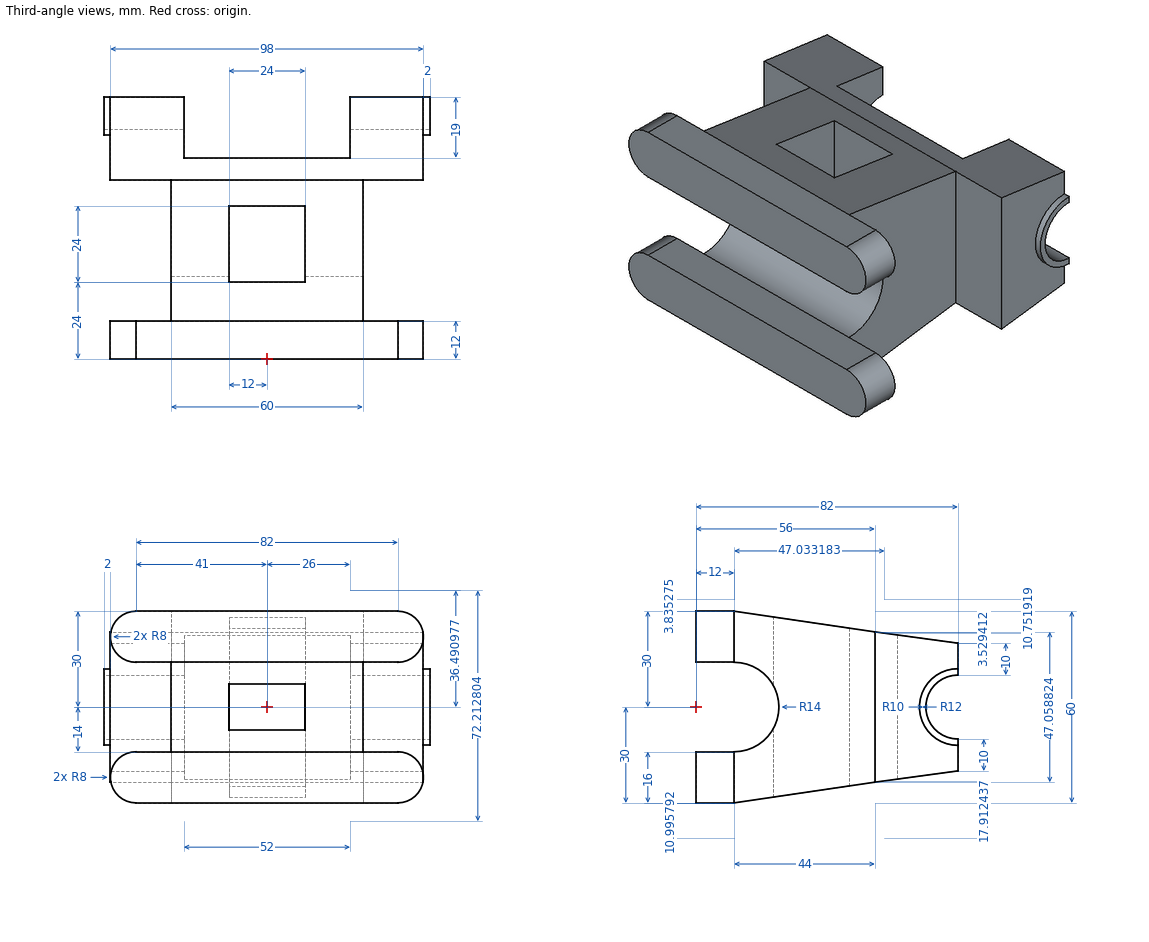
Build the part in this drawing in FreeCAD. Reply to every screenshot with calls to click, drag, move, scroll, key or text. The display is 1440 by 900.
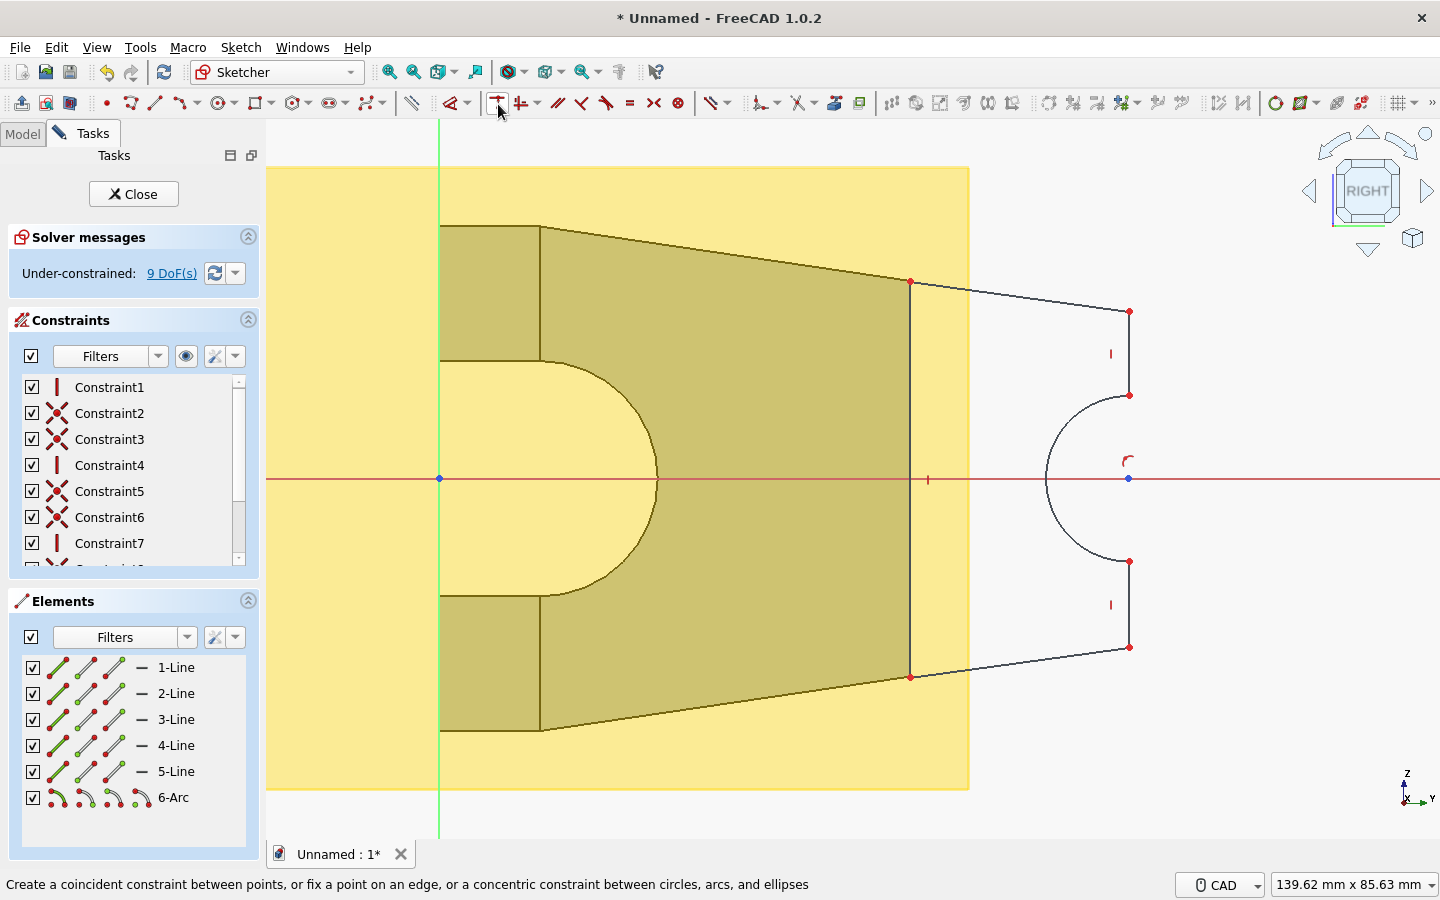
click(450, 104)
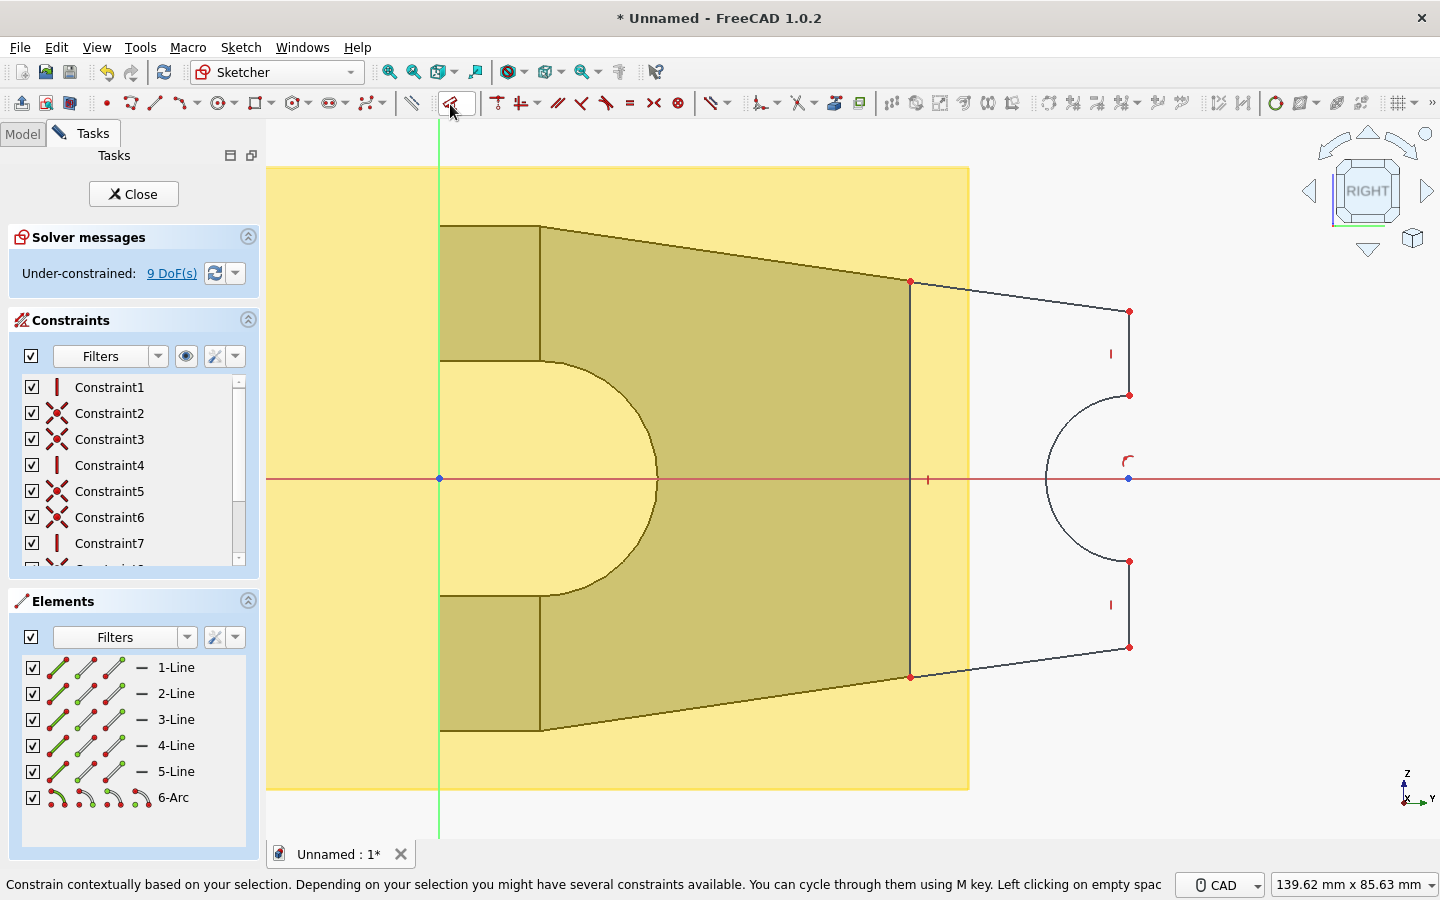
click(1062, 430)
click(1036, 411)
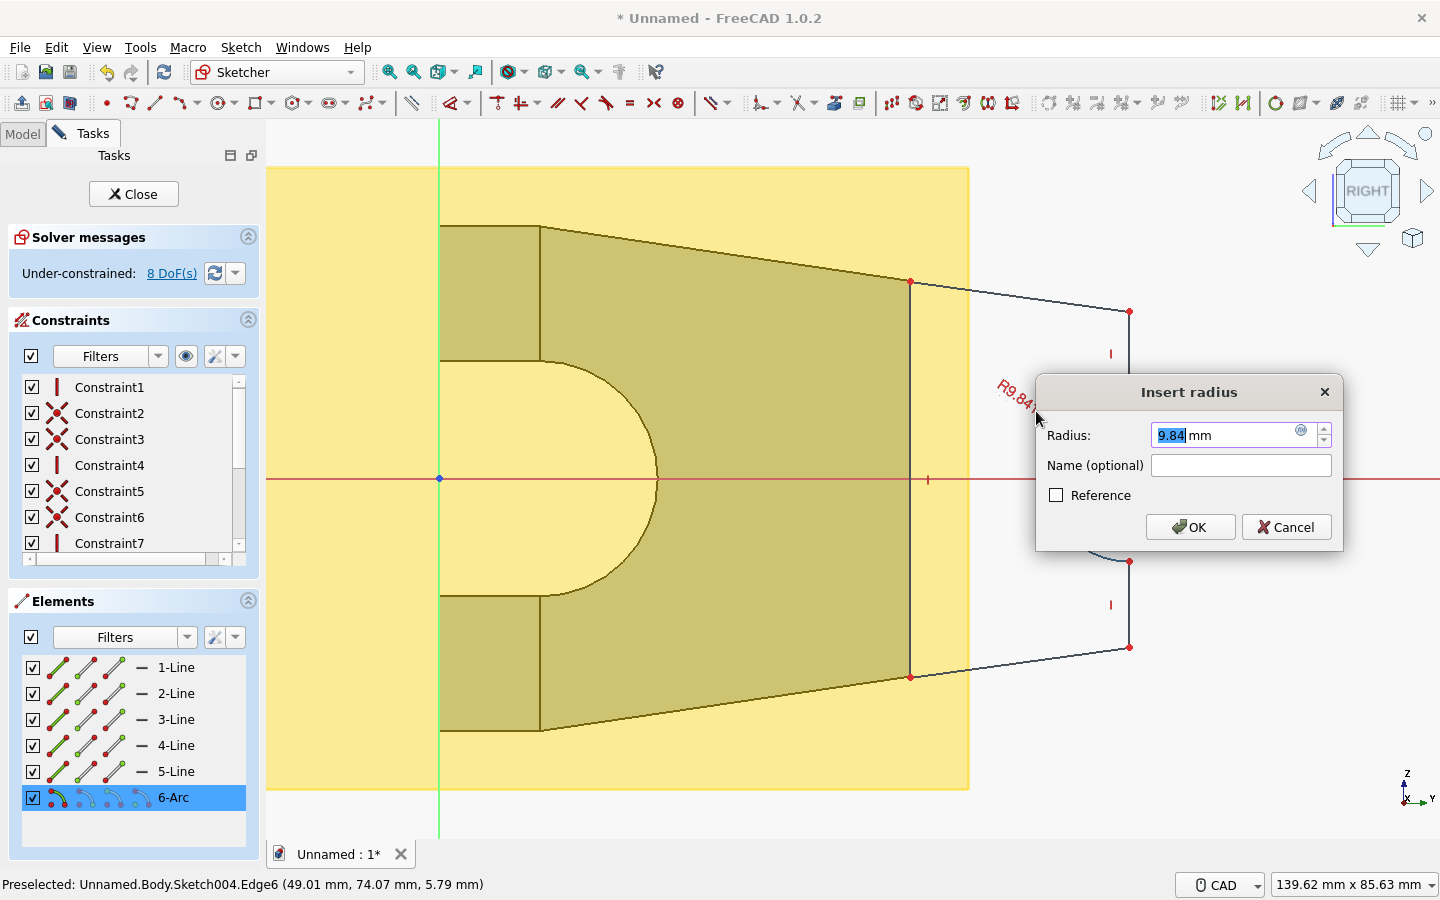
text(10)
key(Return)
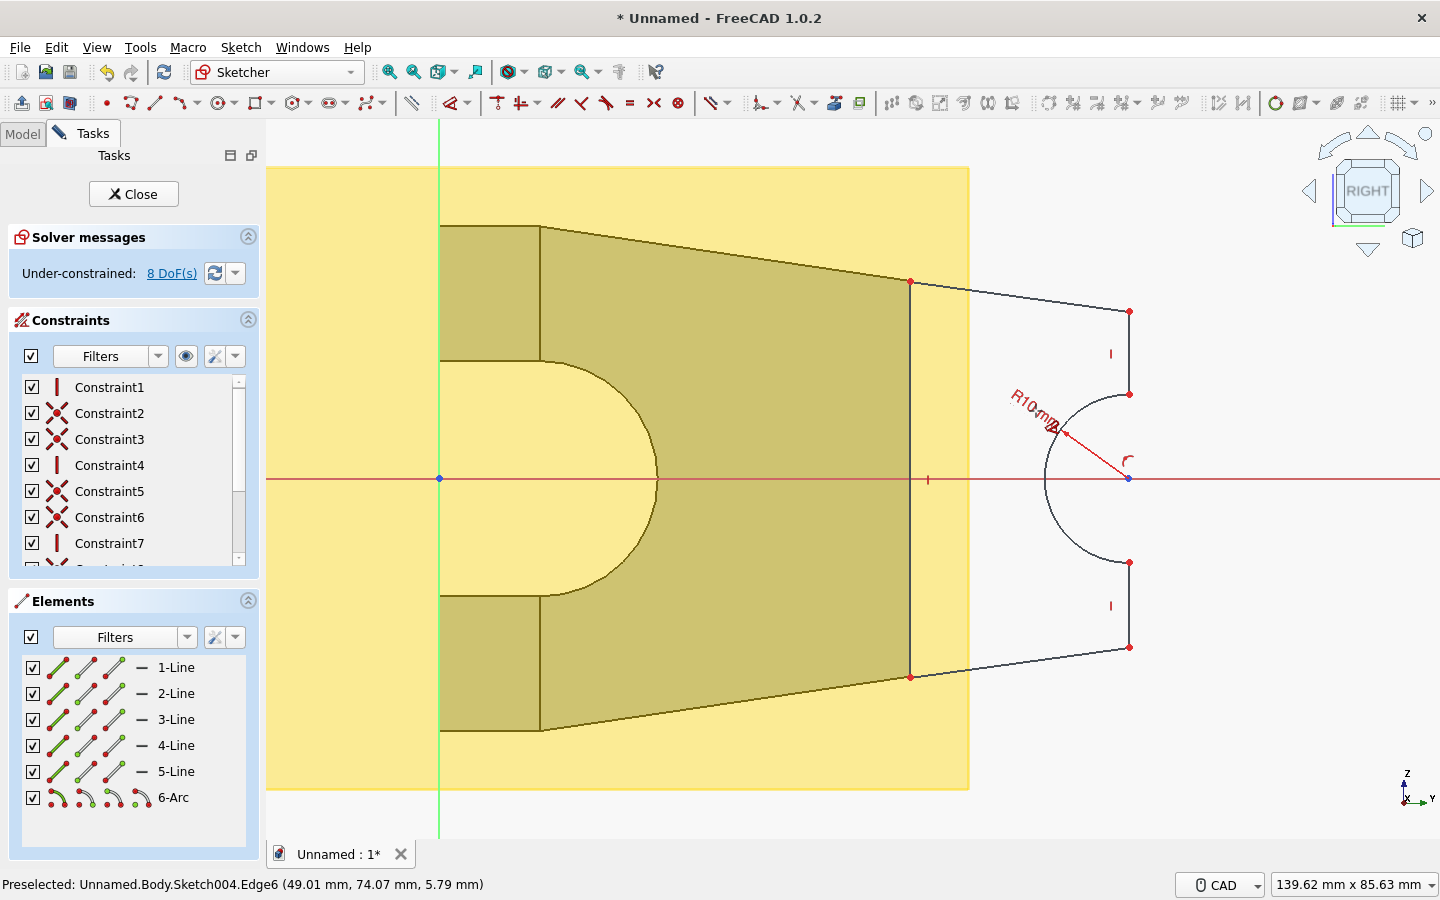
click(1129, 370)
click(1163, 353)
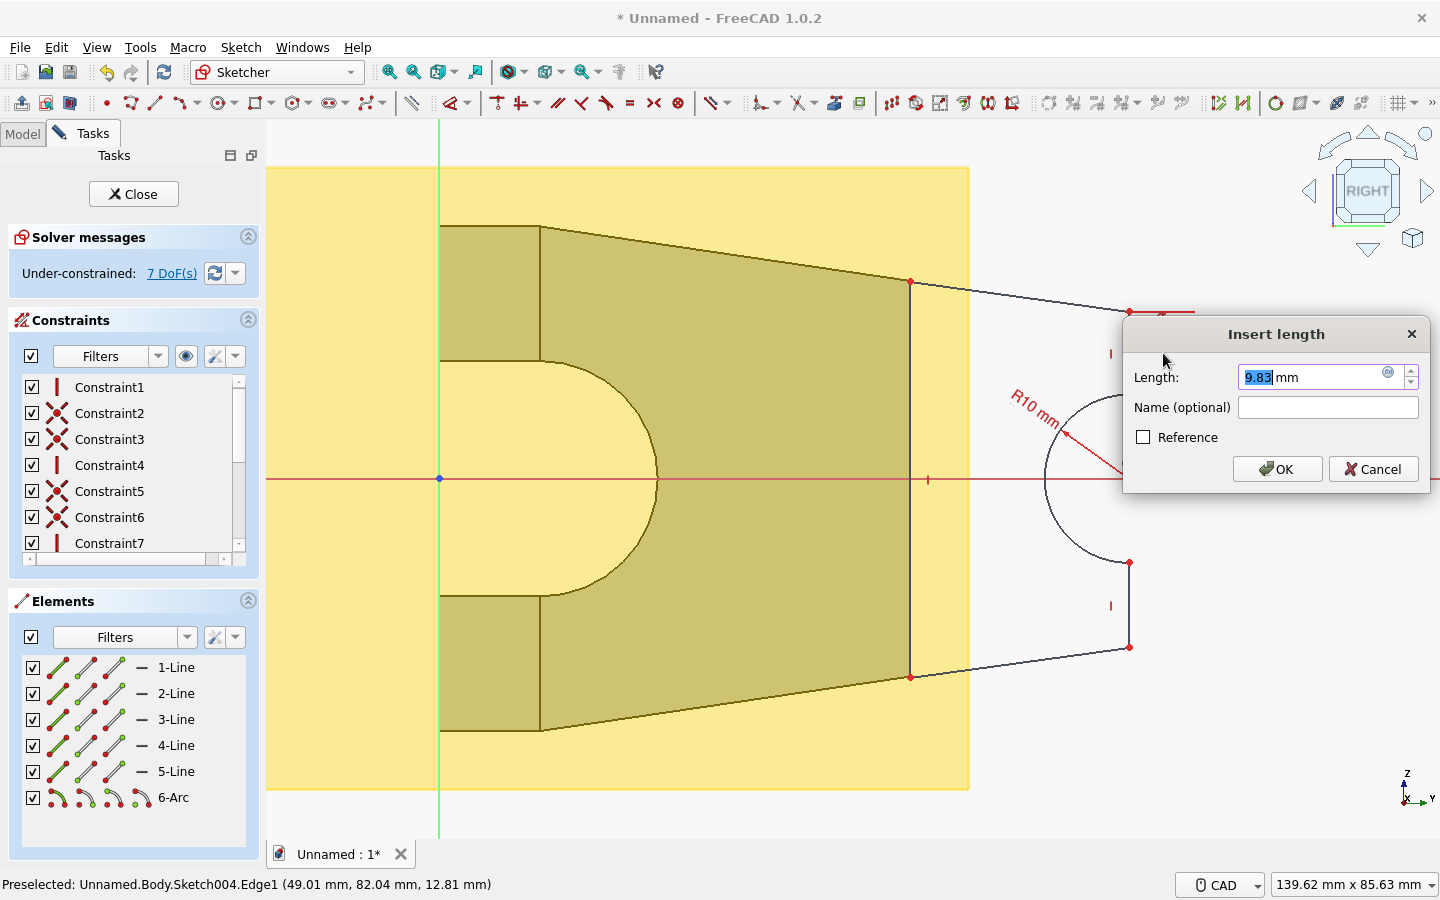
text(10)
key(Return)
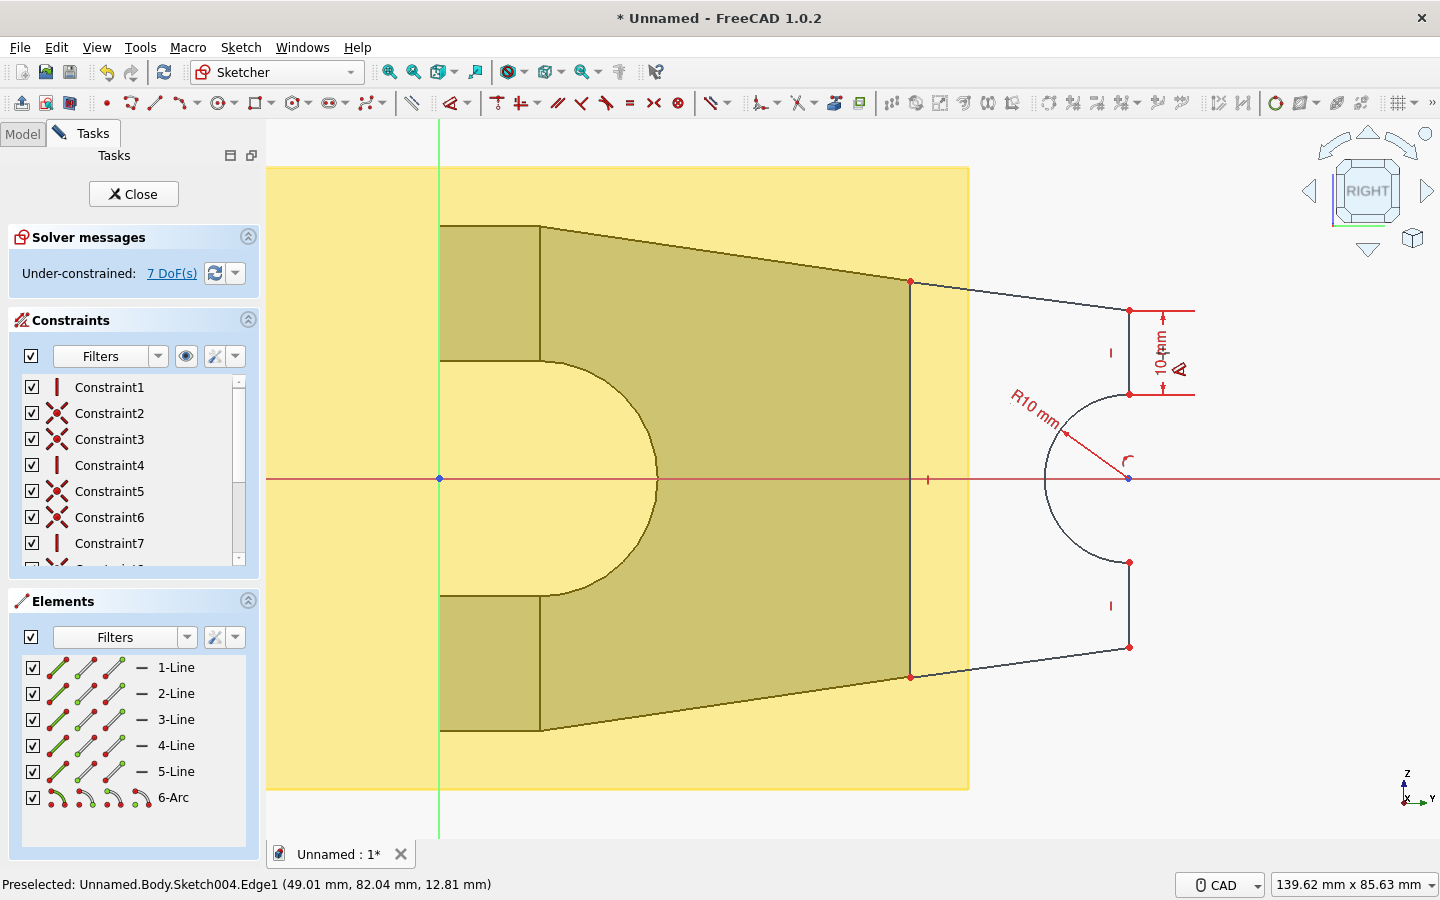
click(1129, 622)
click(1163, 605)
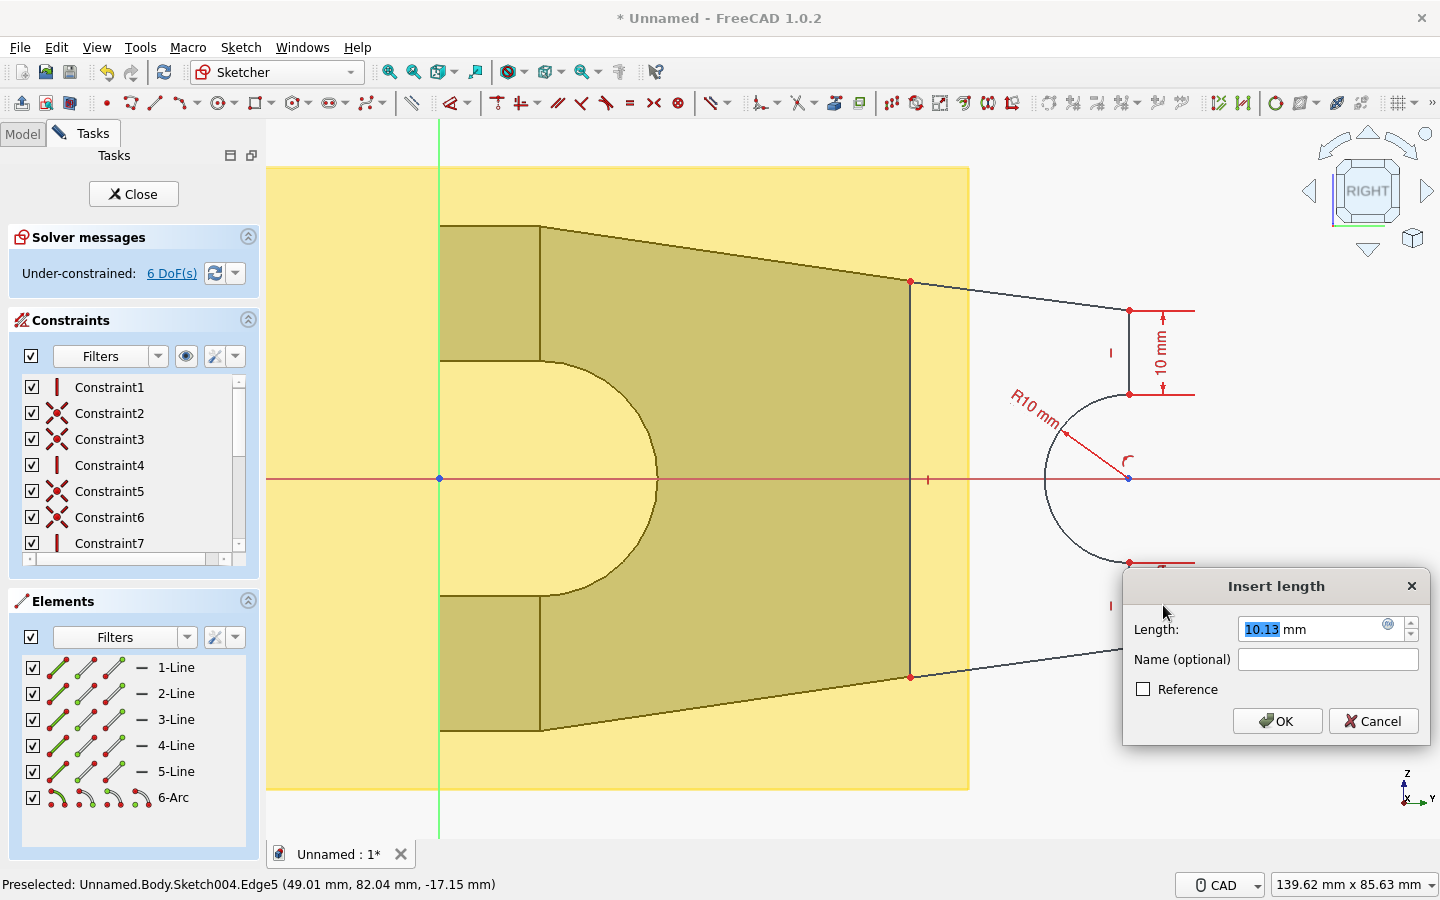
text(10)
key(Return)